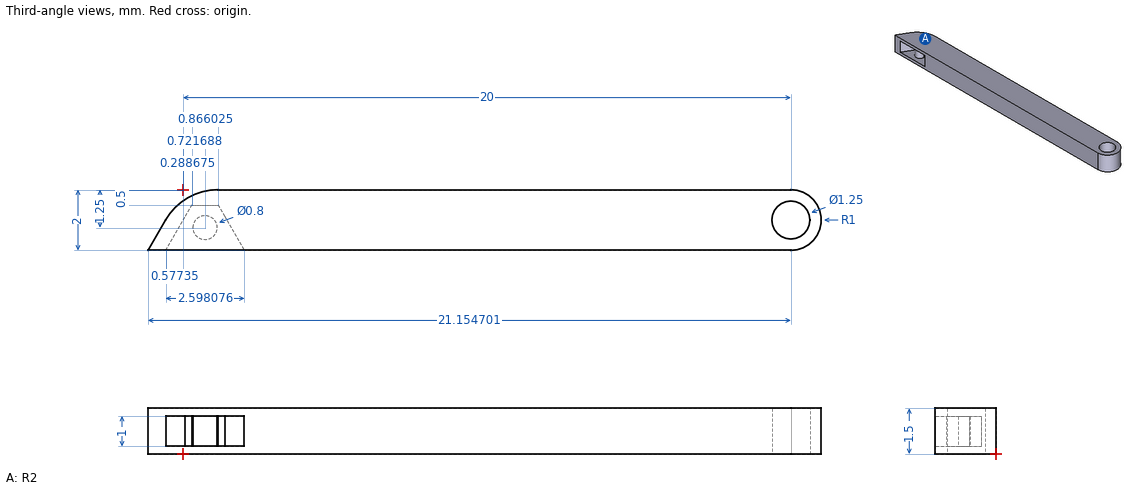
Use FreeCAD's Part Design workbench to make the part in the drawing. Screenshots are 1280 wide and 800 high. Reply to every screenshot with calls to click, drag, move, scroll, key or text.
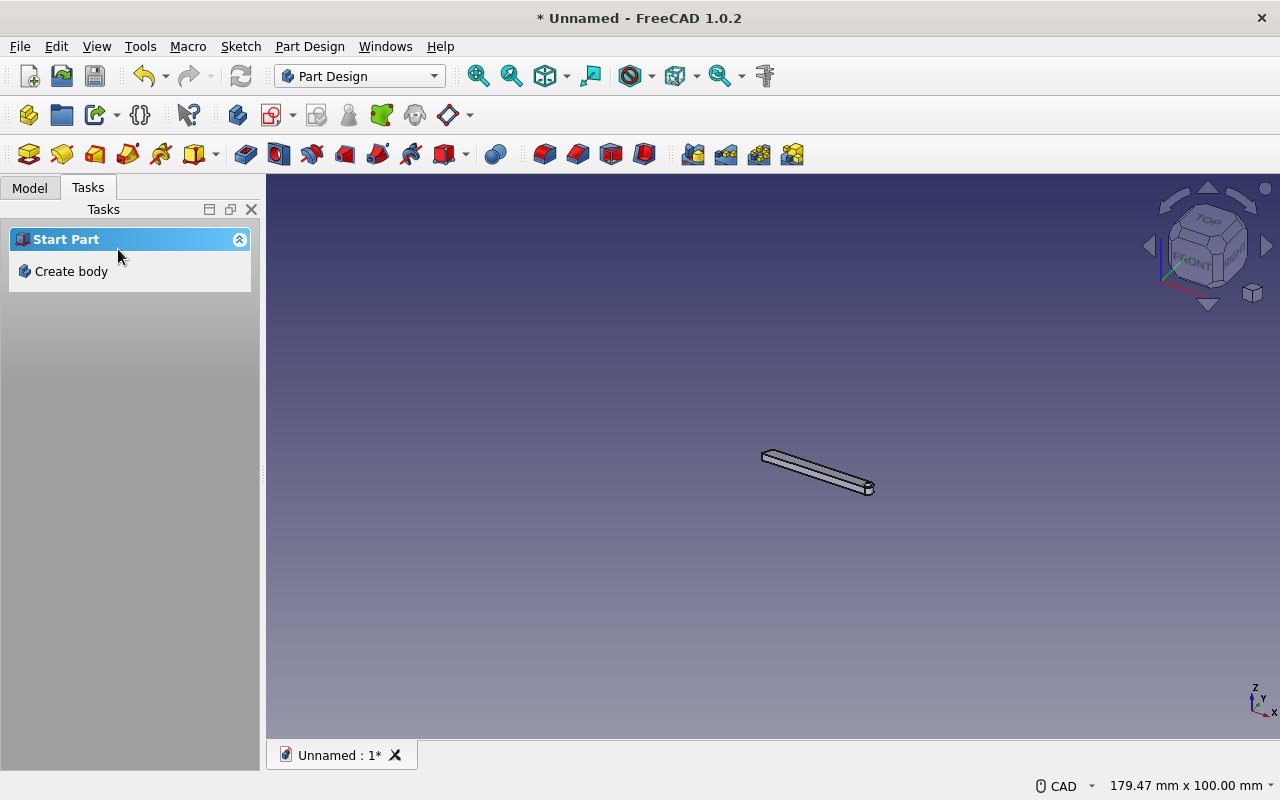
key(v)
key(f)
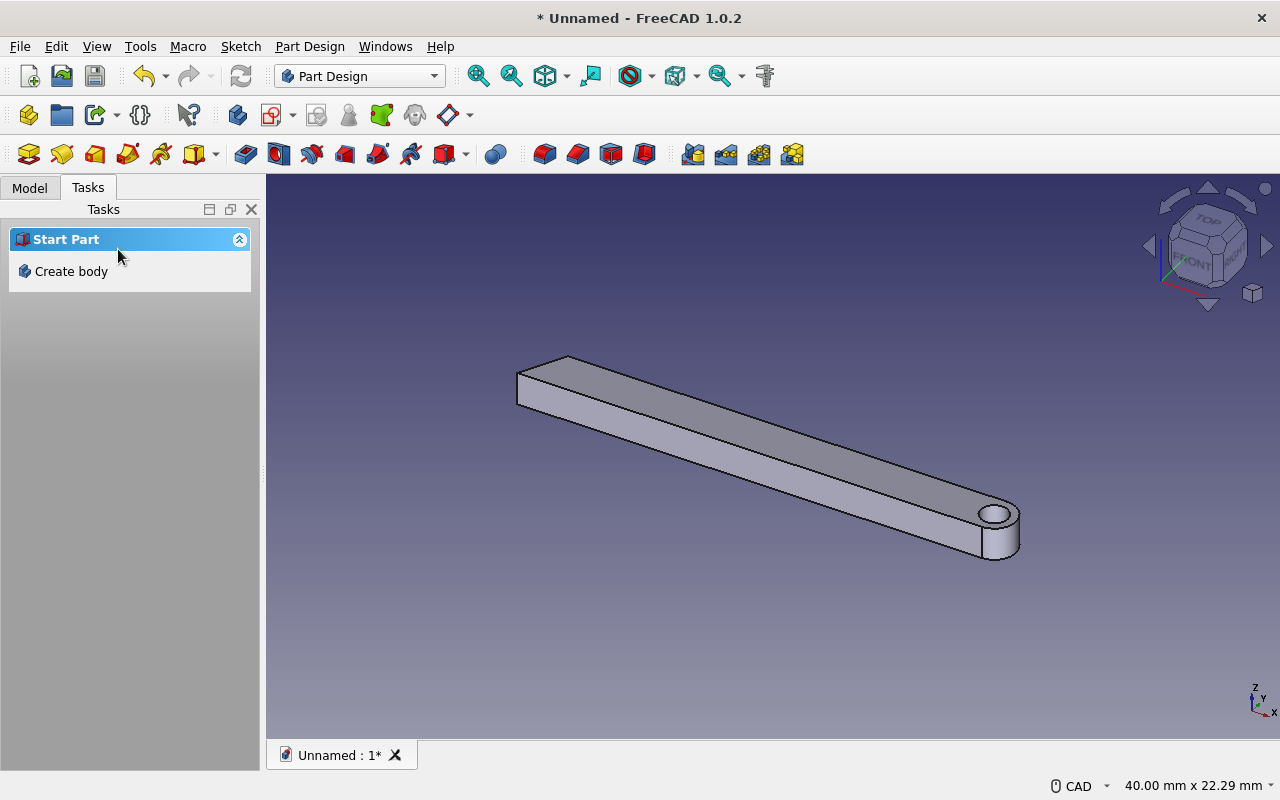
click(30, 188)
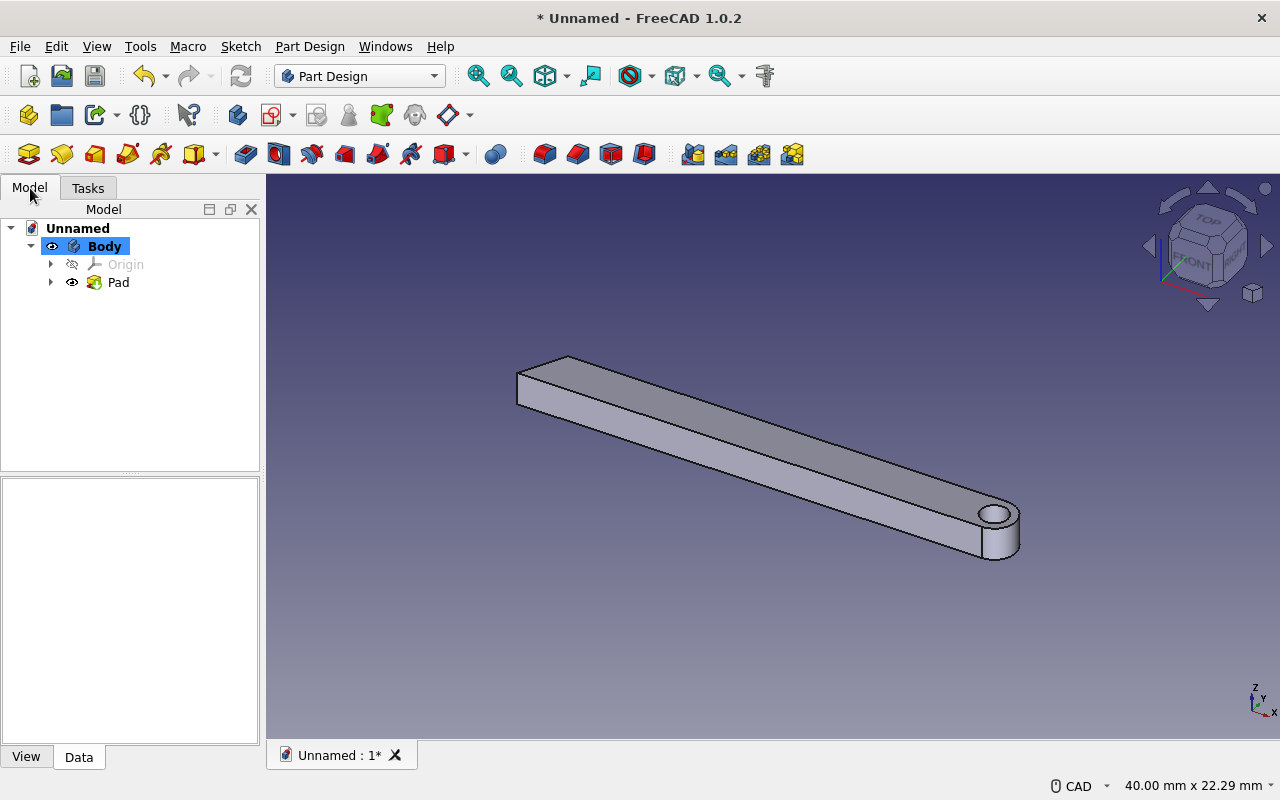
click(51, 264)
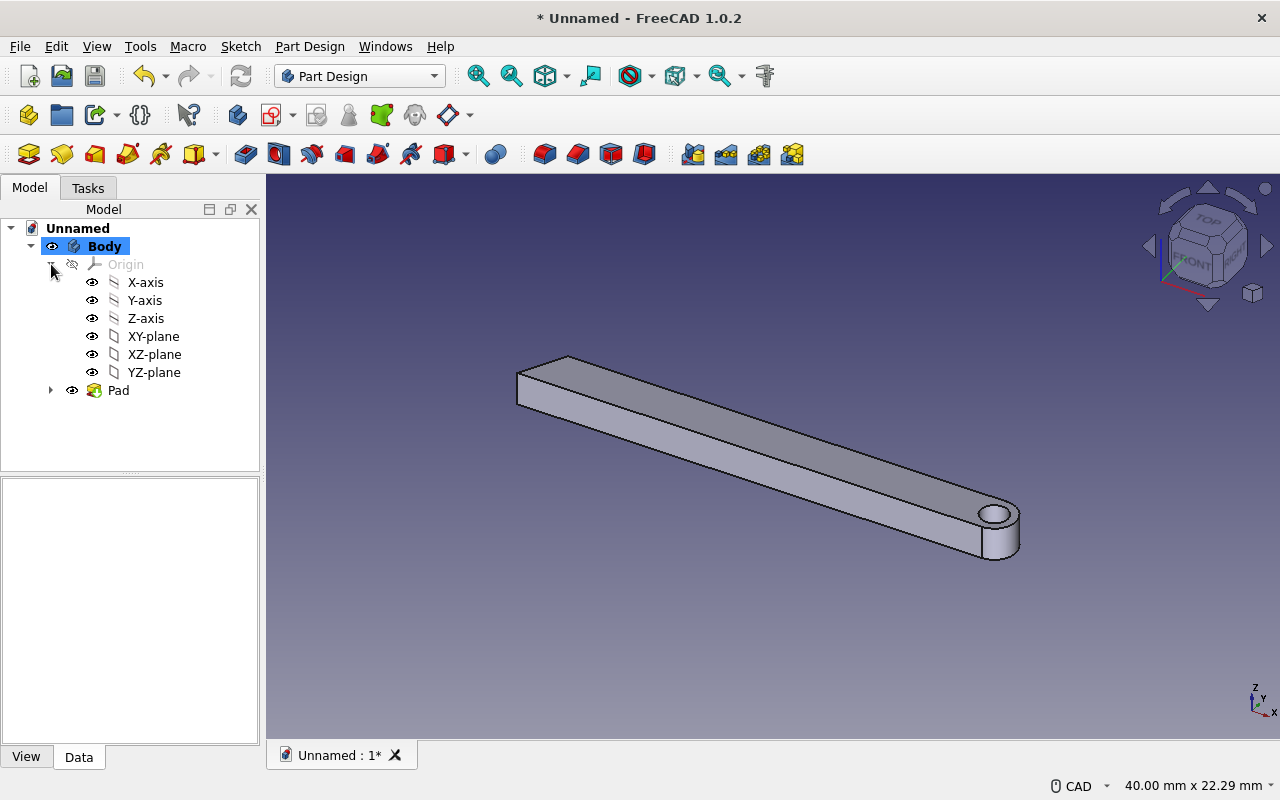
click(137, 336)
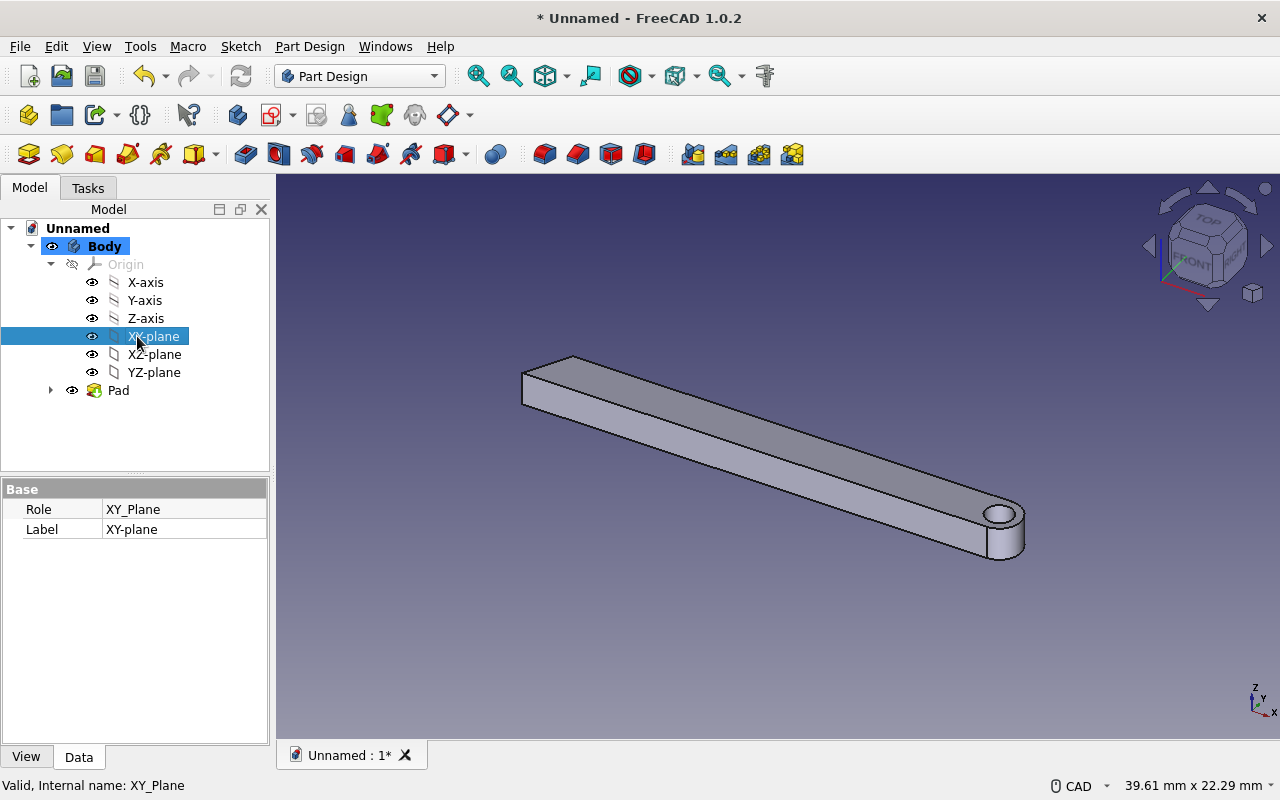
click(448, 116)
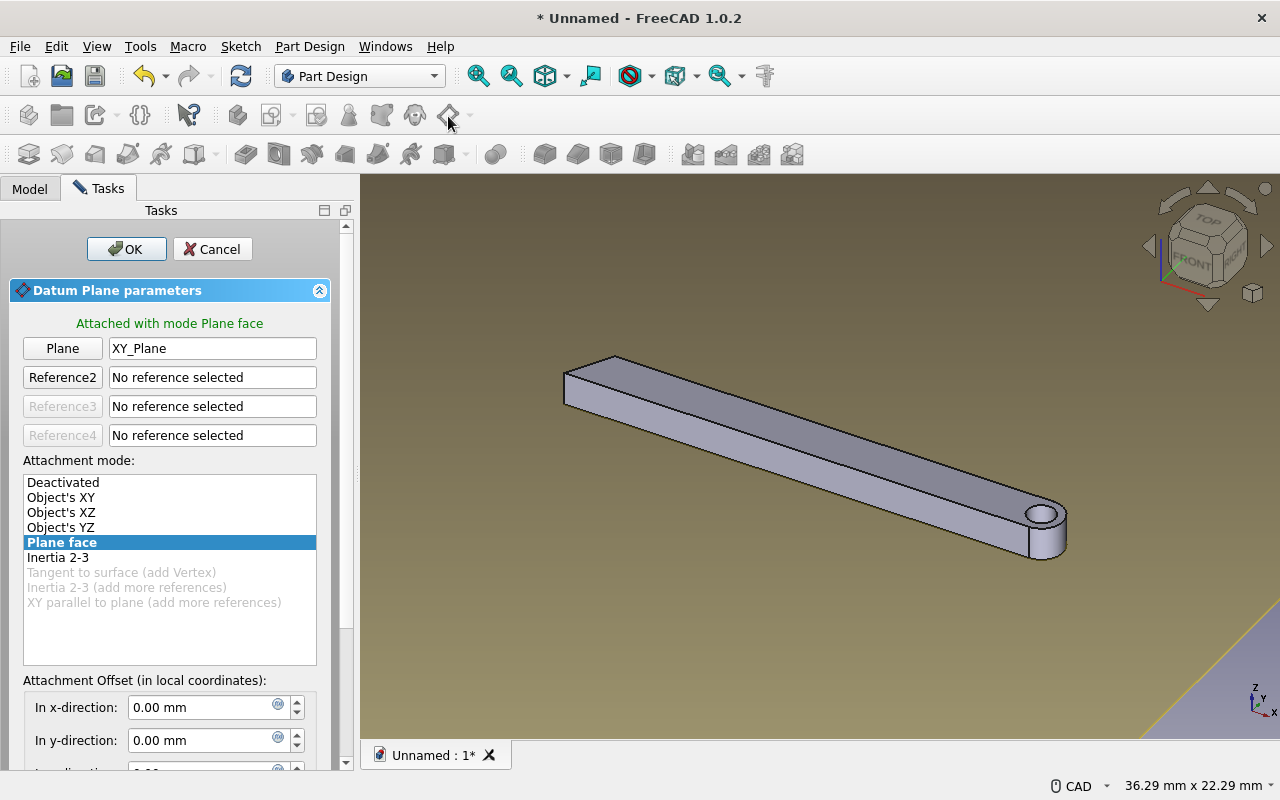
scroll(346, 495, down, 2)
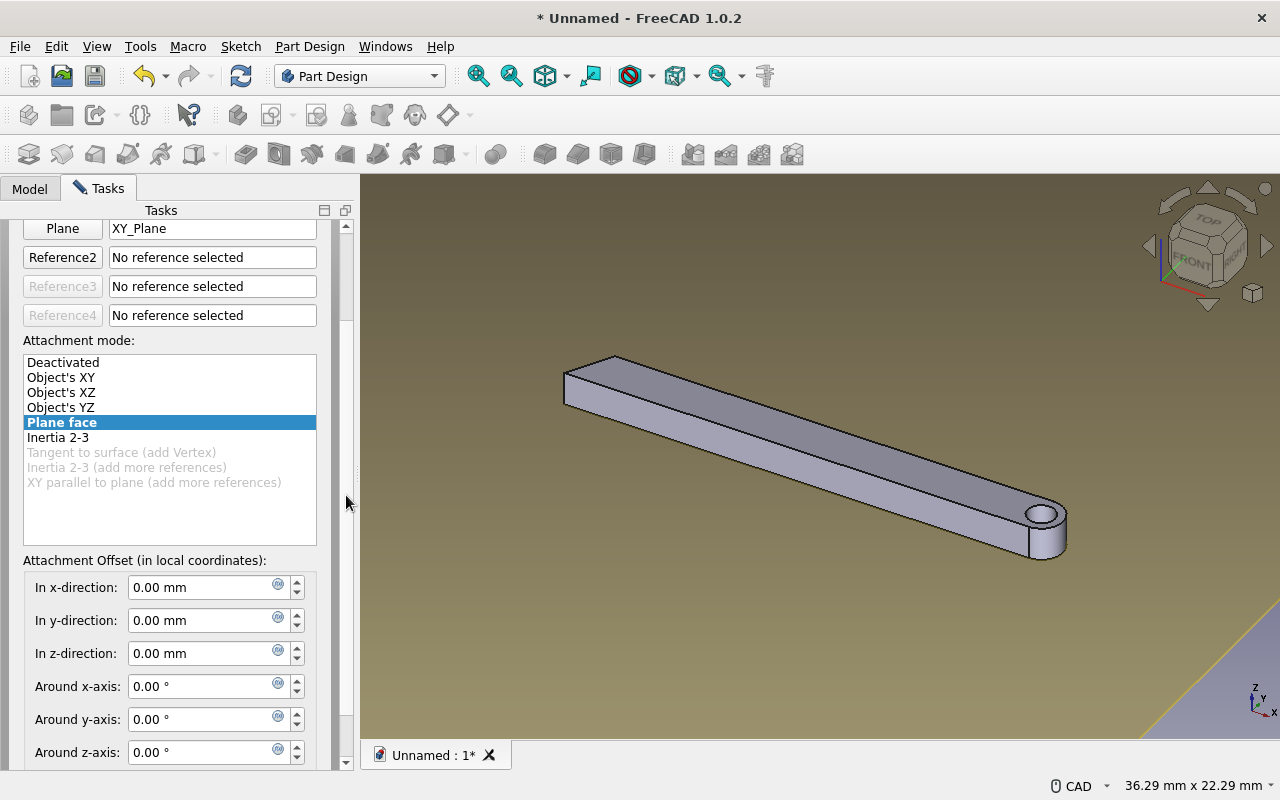
triple_click(210, 654)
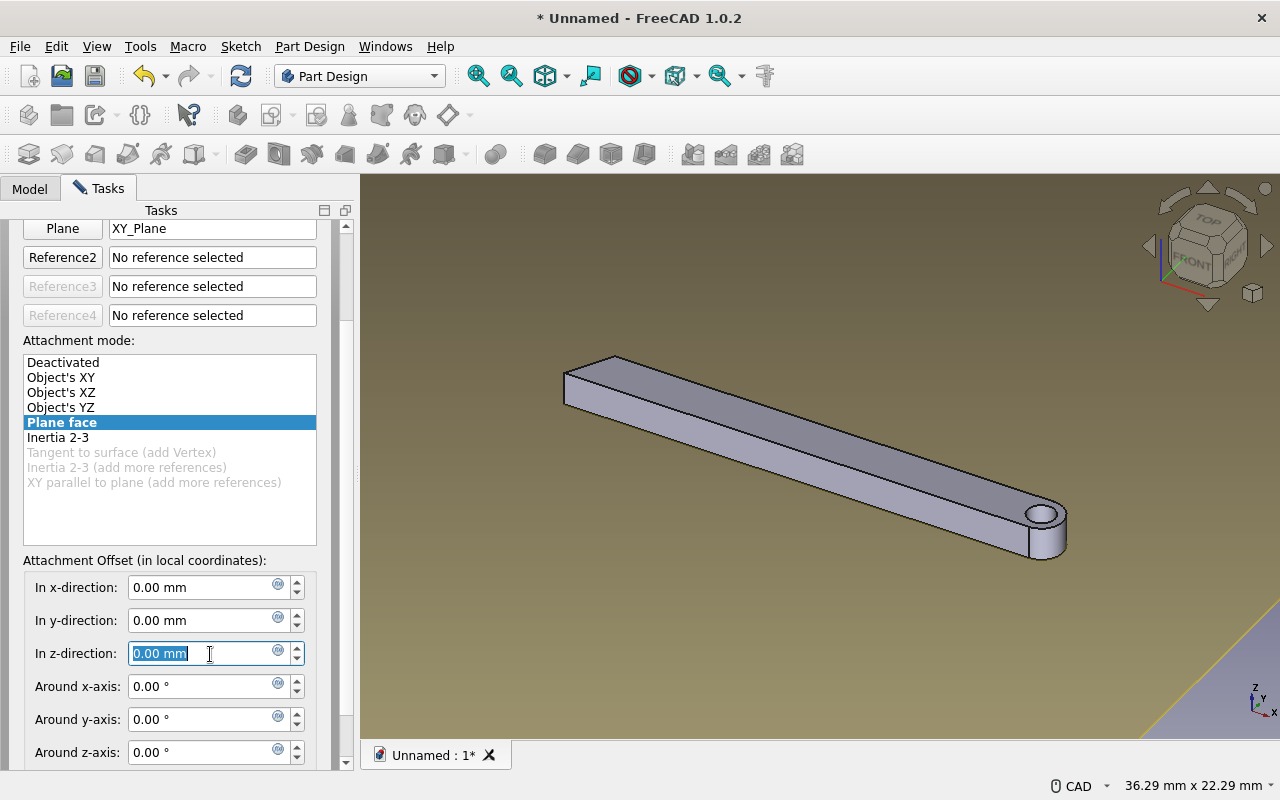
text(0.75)
key(Tab)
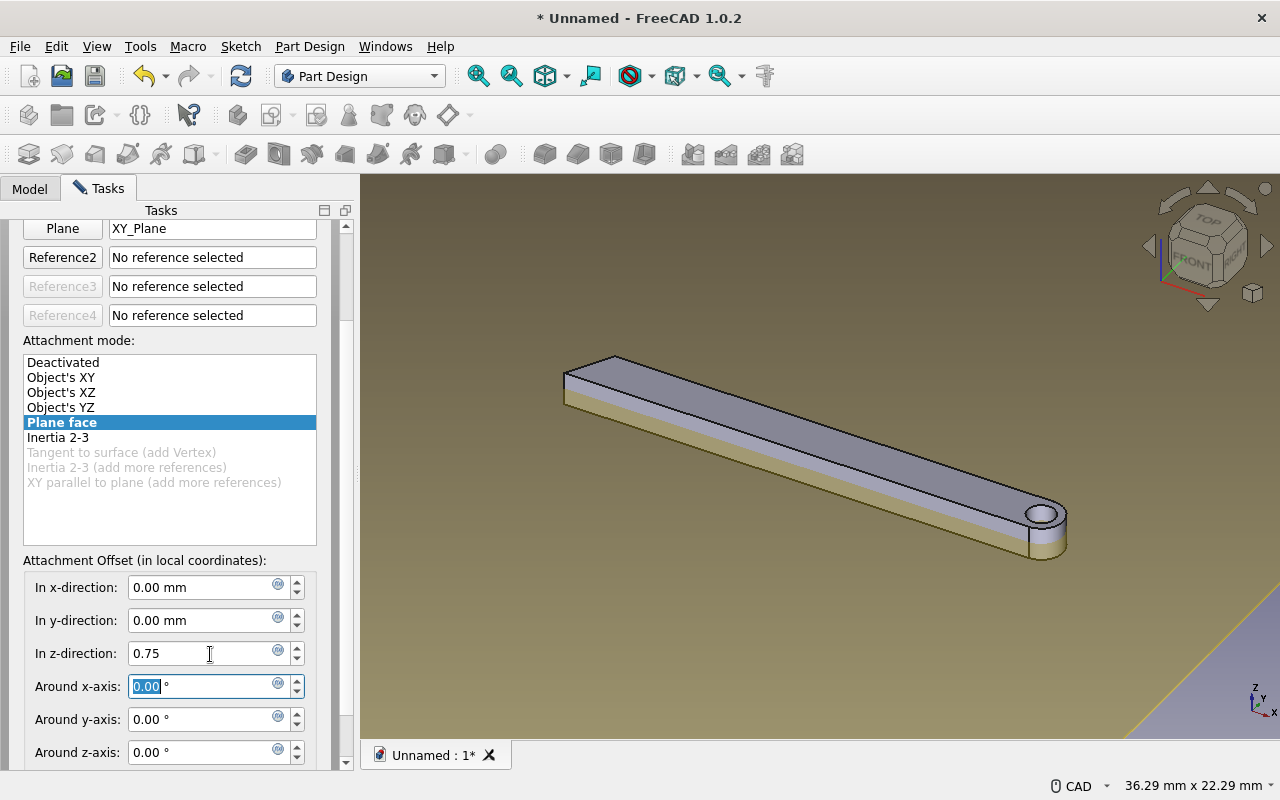
scroll(346, 495, up, 3)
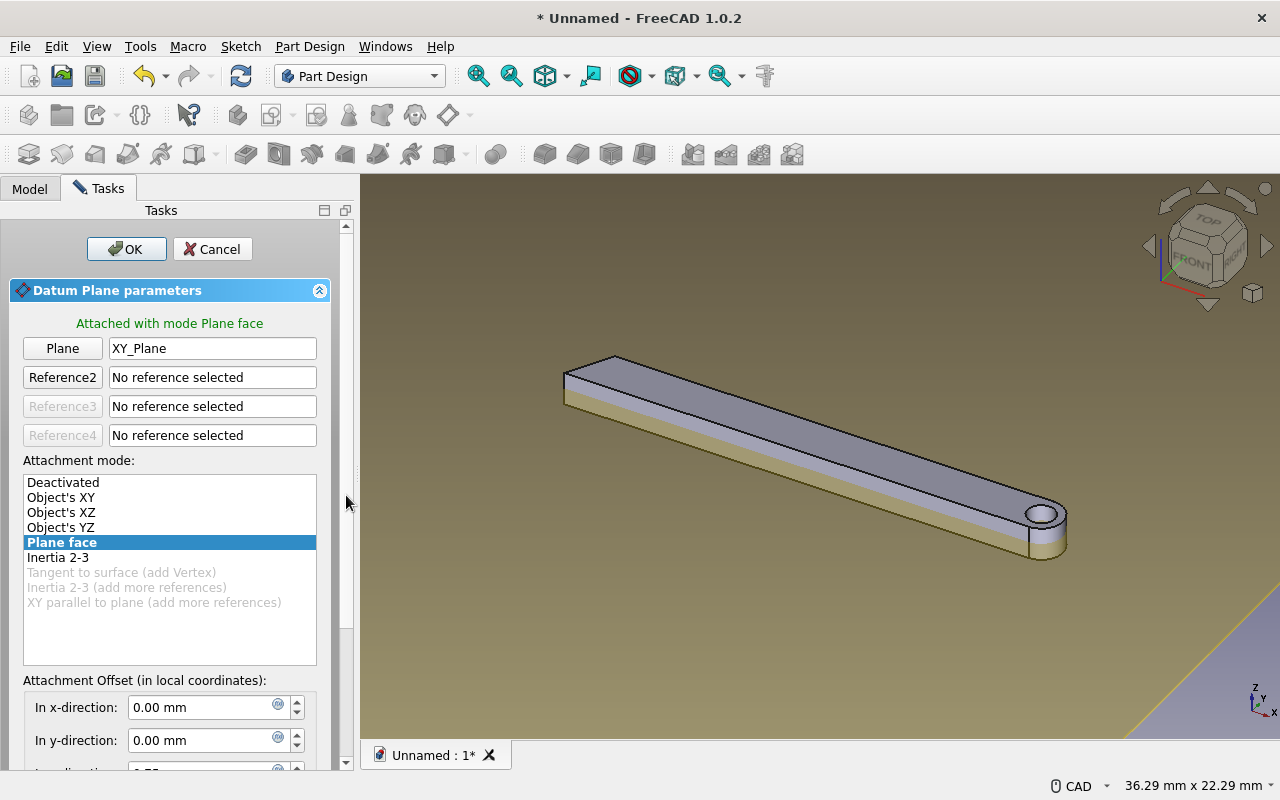
click(127, 249)